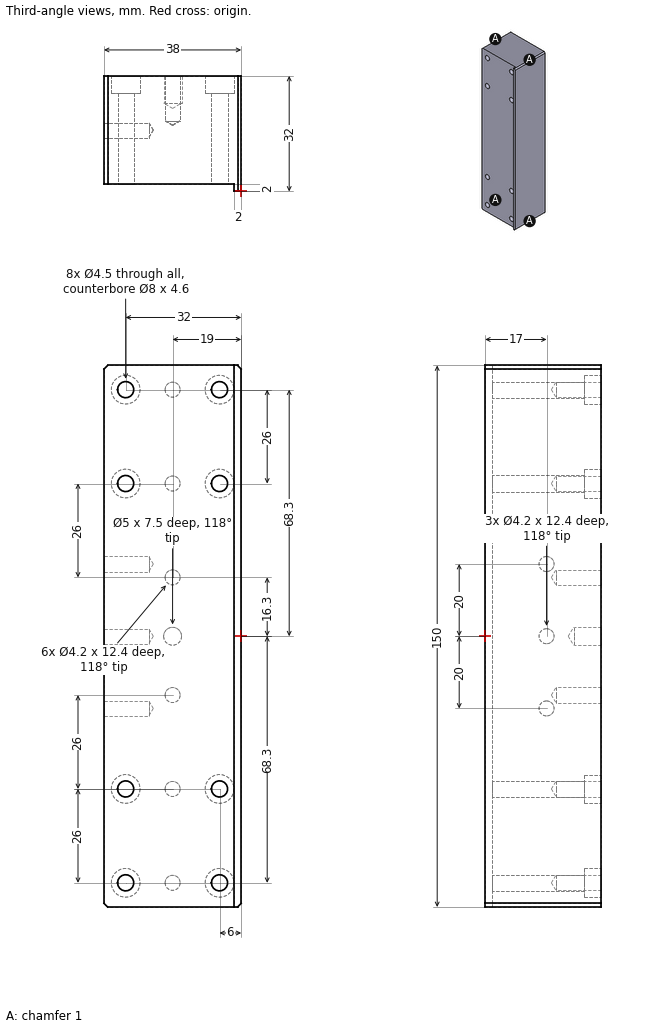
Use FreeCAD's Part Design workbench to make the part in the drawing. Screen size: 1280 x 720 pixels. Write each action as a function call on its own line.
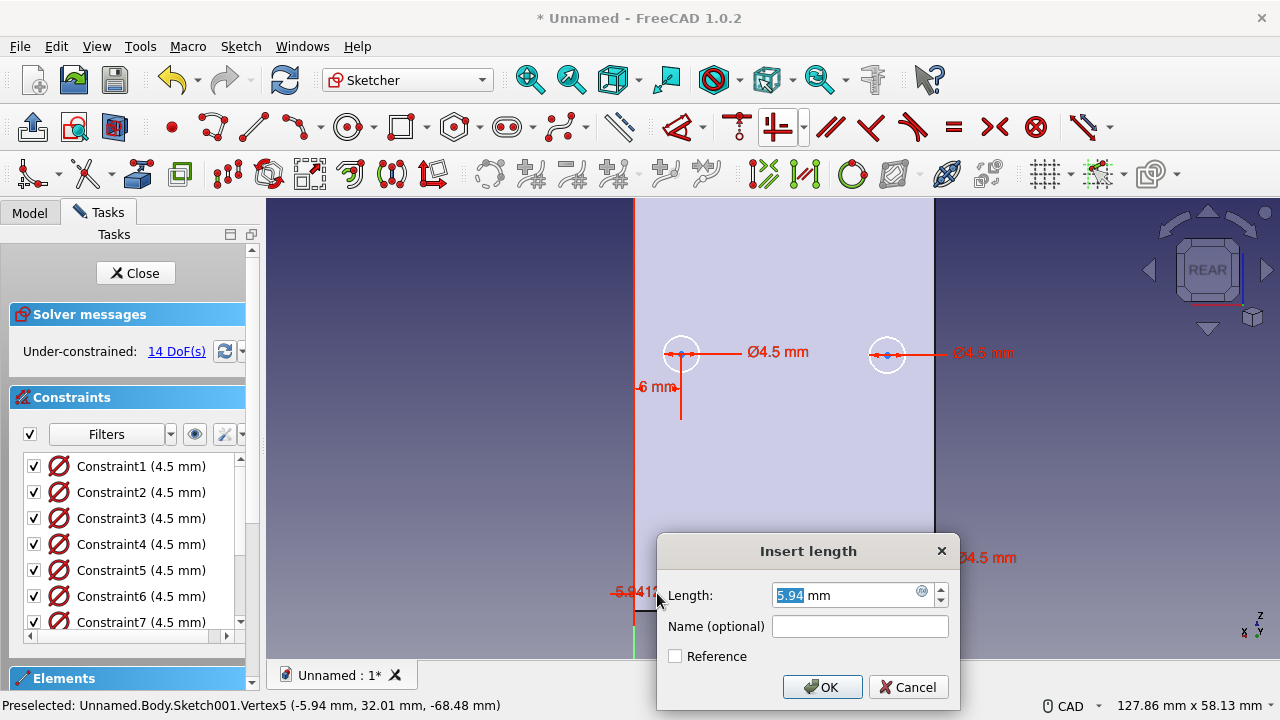
text(6)
key(Return)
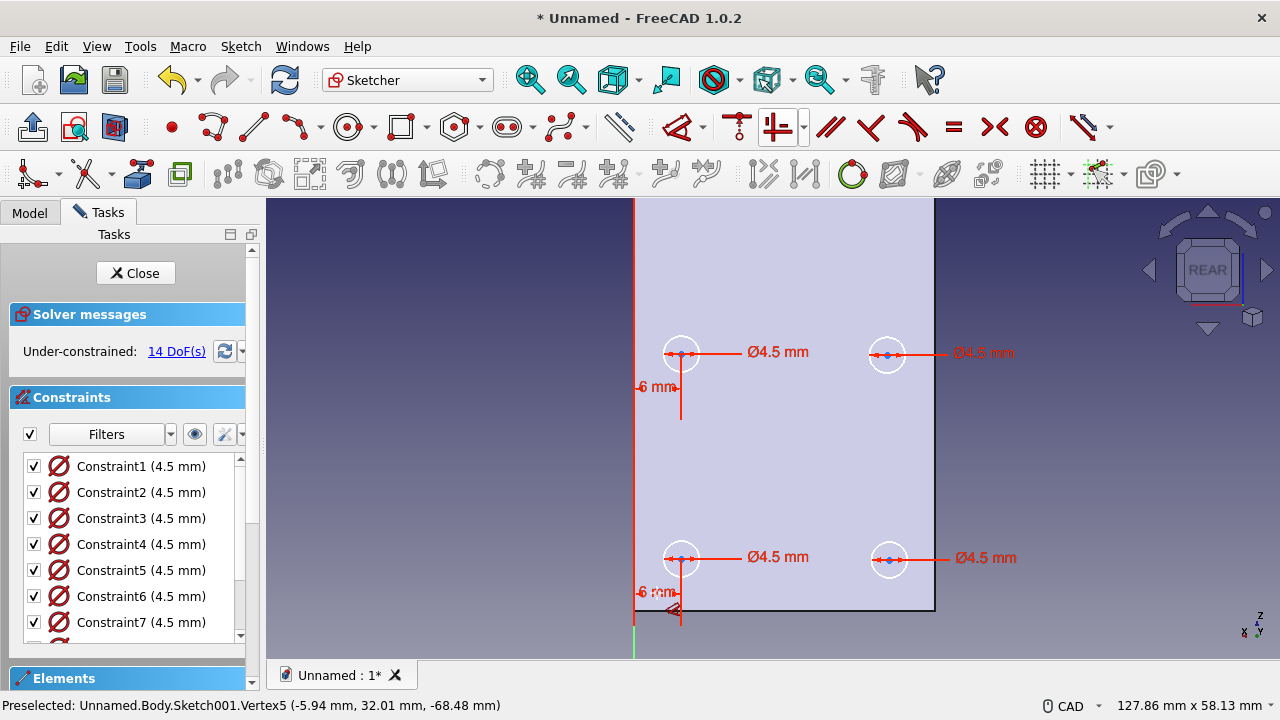
scroll(683, 564, down, 7)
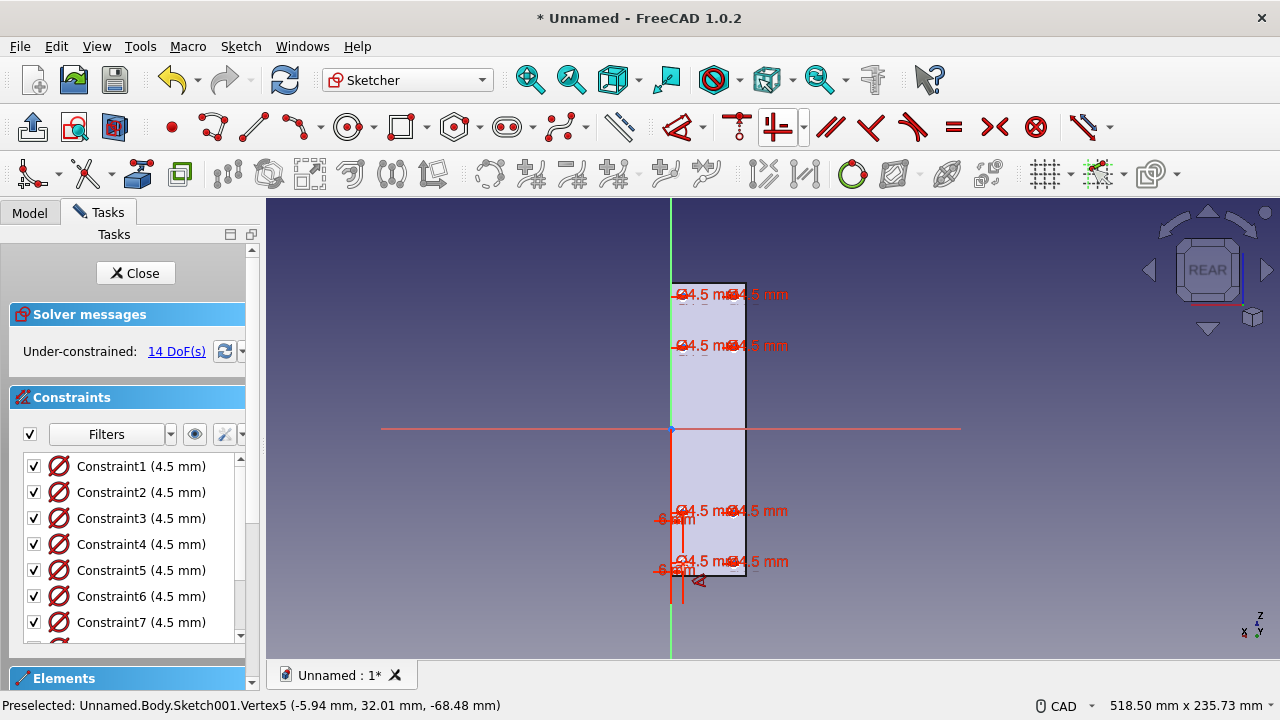
scroll(683, 297, up, 7)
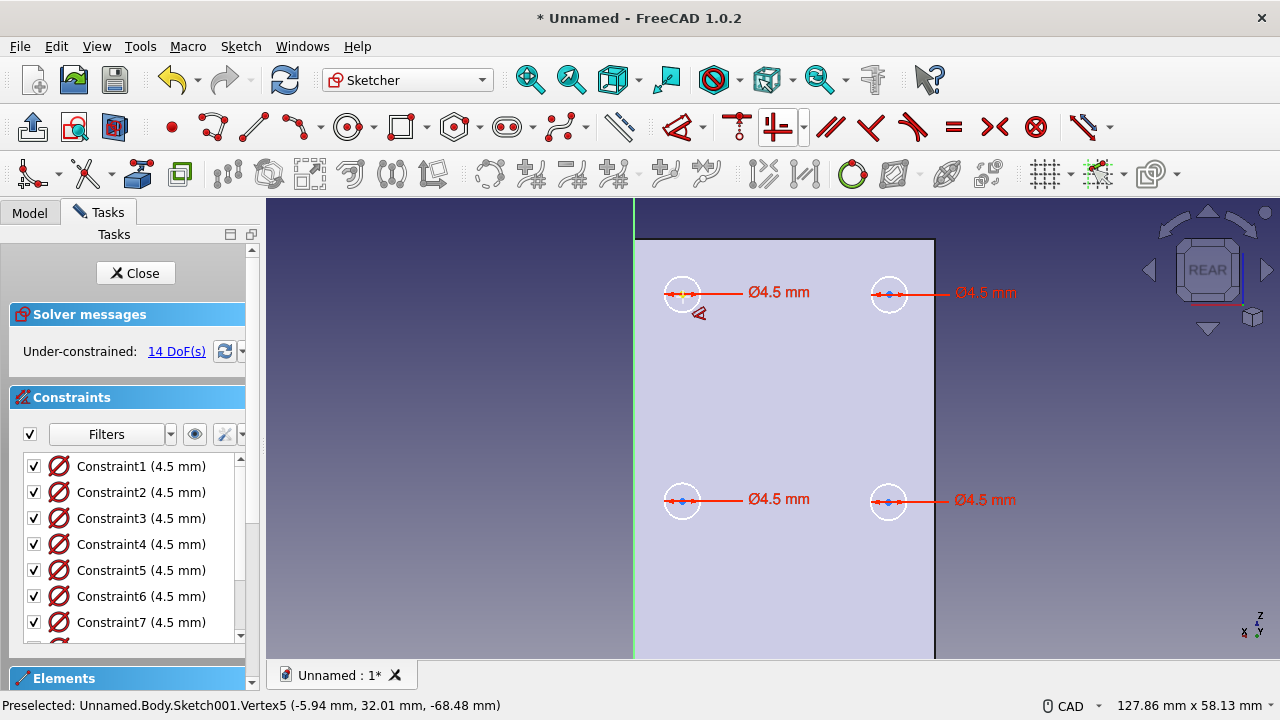
click(682, 294)
click(658, 260)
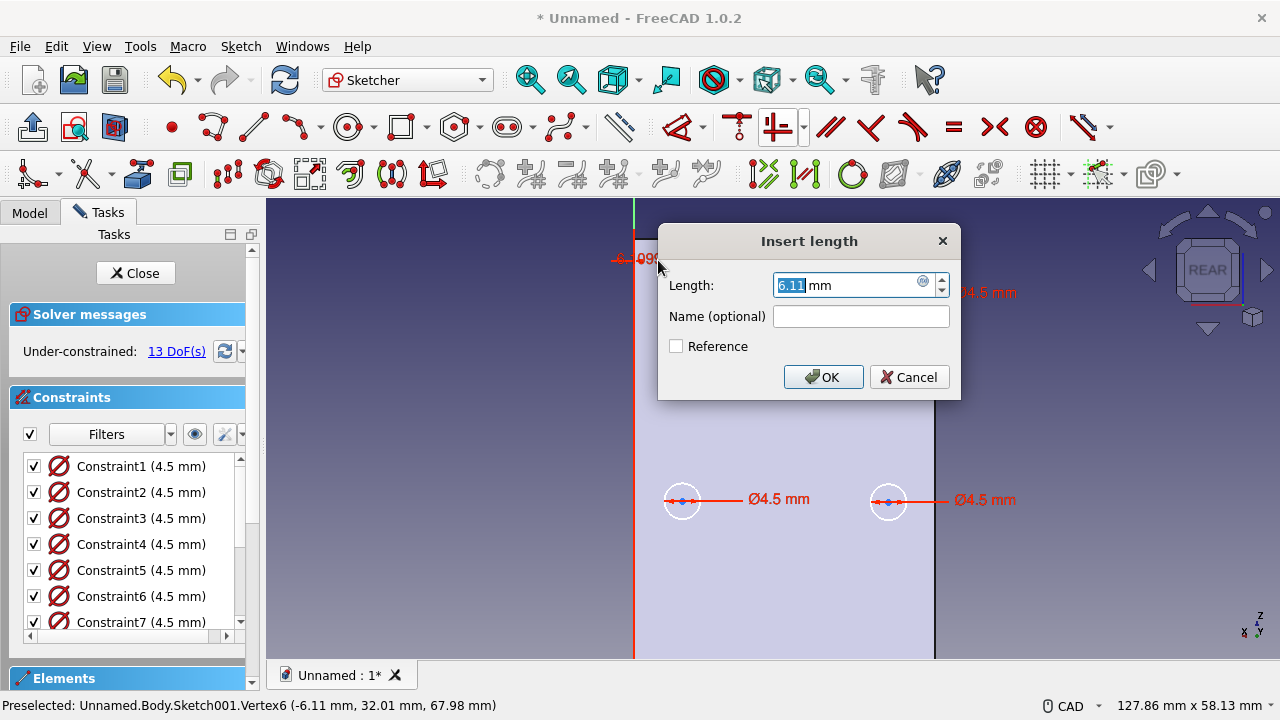
text(6)
key(Return)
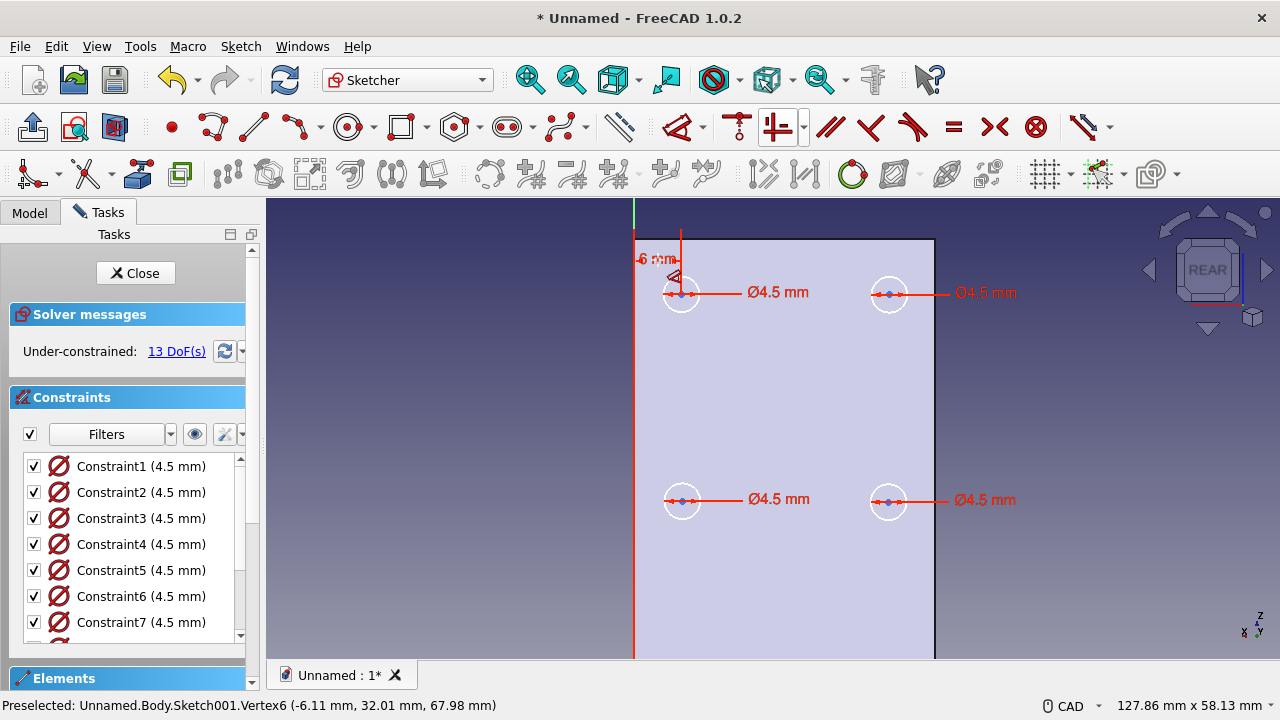
click(682, 501)
click(658, 467)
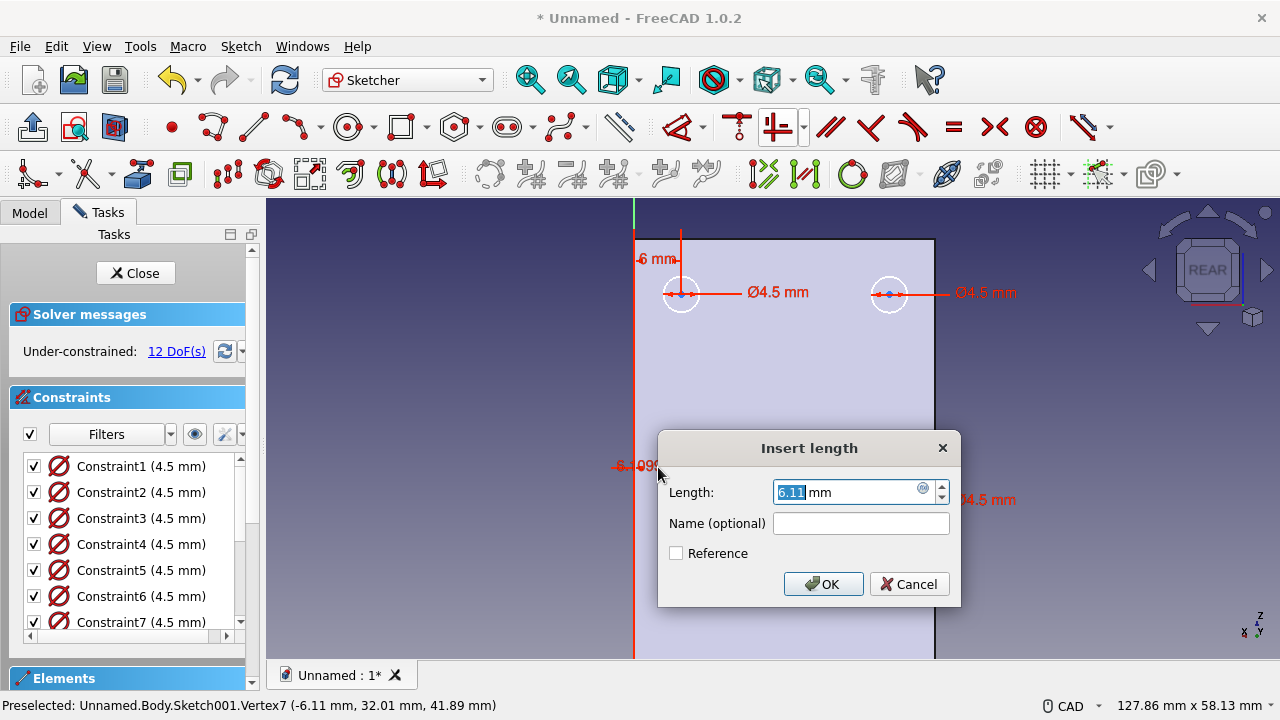
text(6)
key(Return)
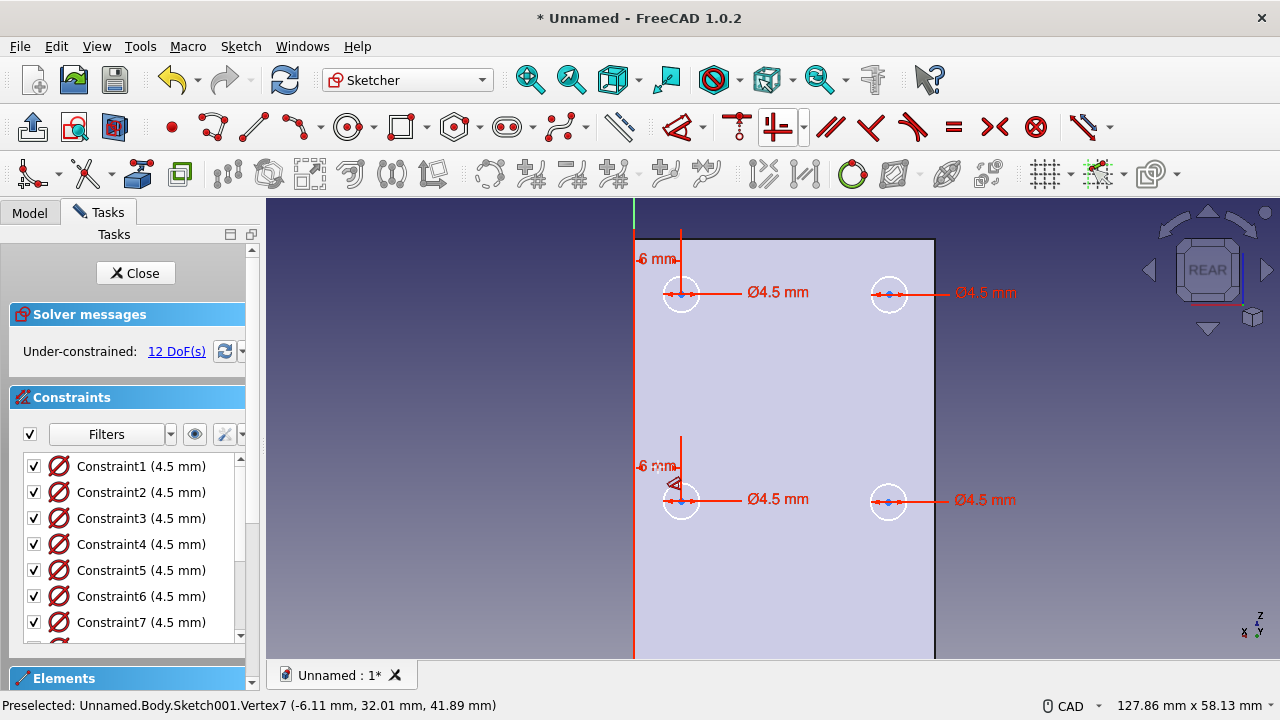
scroll(683, 296, down, 7)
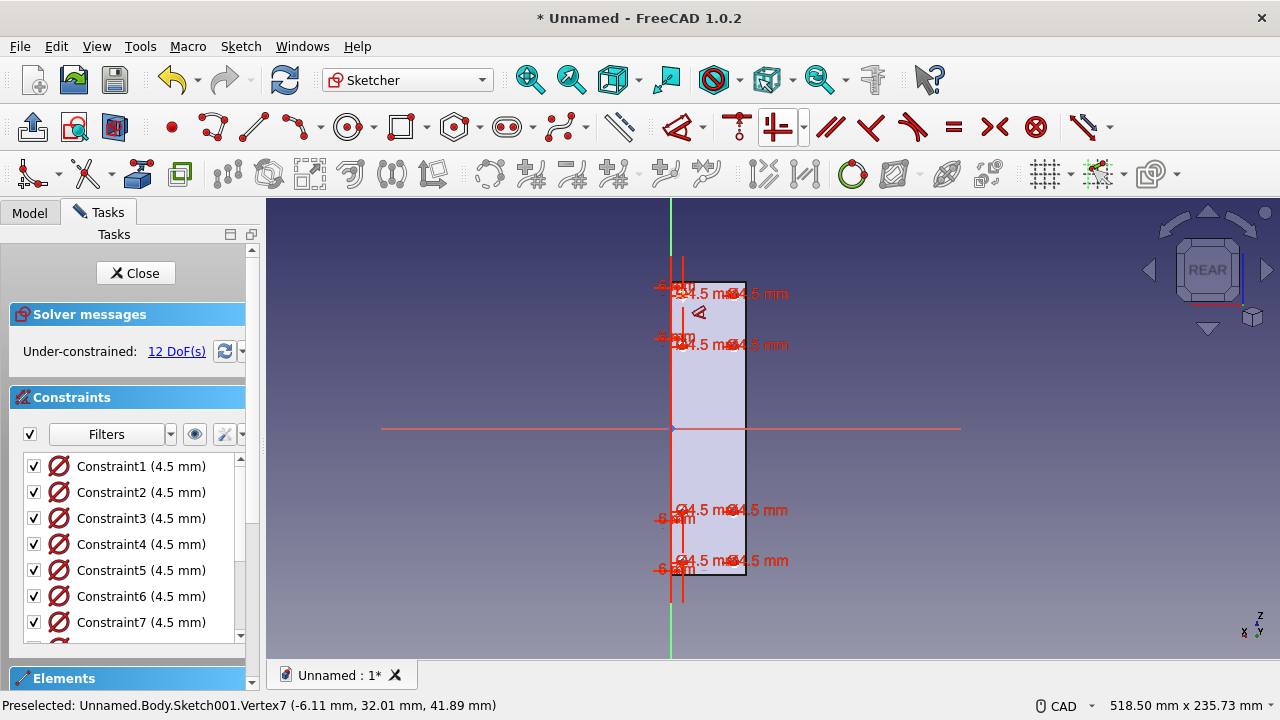
click(734, 296)
click(703, 262)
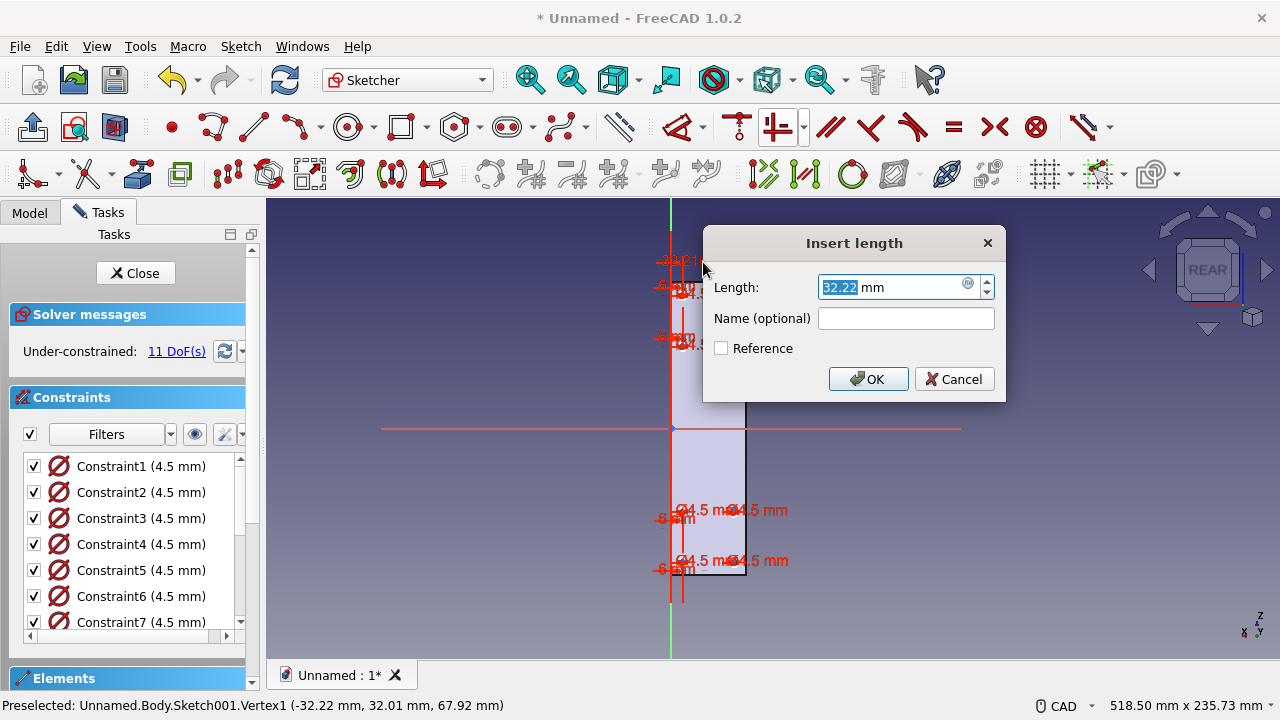
text(32)
key(Return)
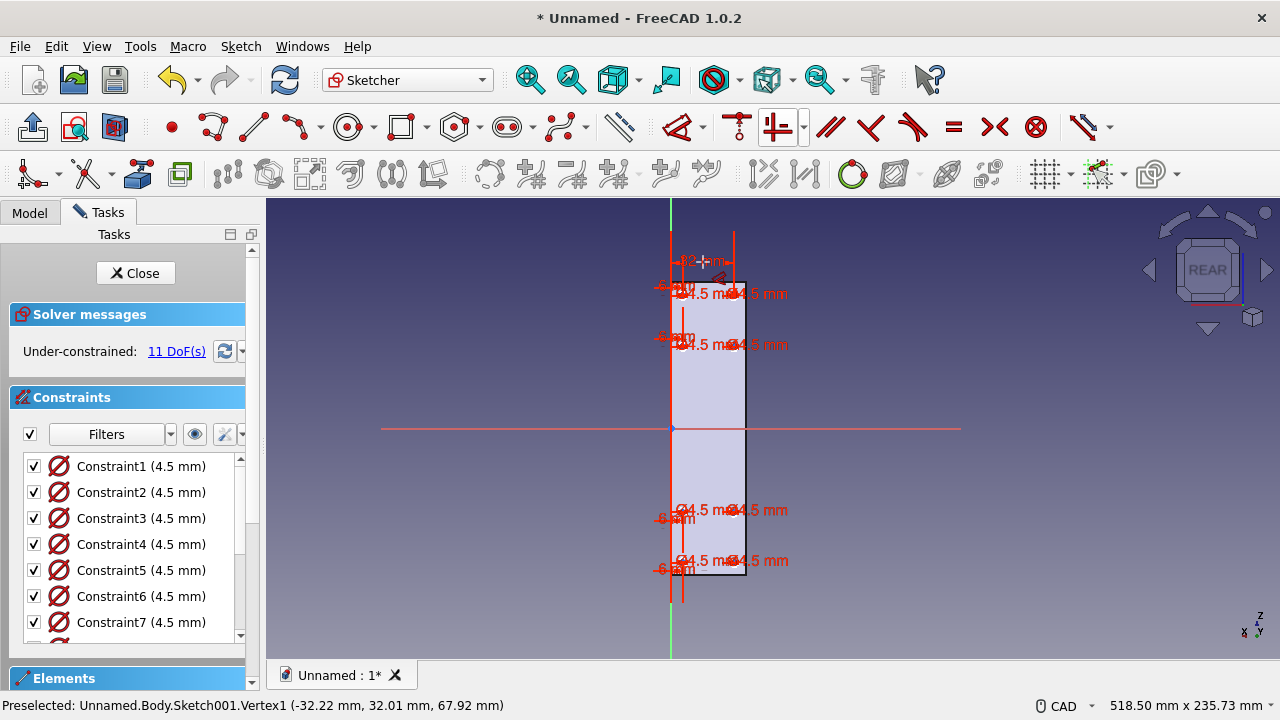
click(734, 563)
click(703, 597)